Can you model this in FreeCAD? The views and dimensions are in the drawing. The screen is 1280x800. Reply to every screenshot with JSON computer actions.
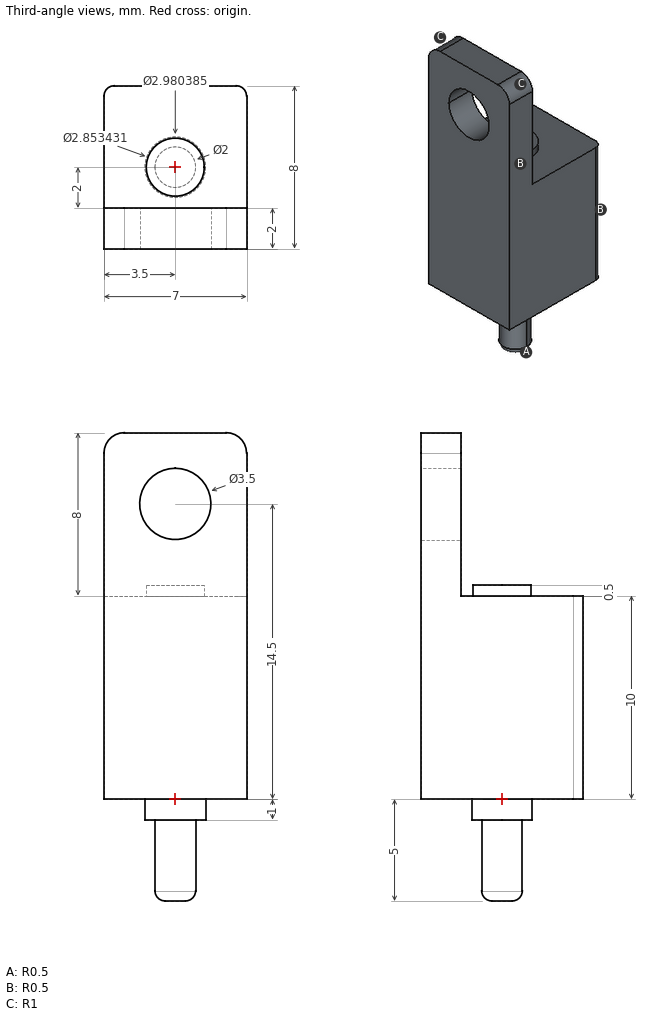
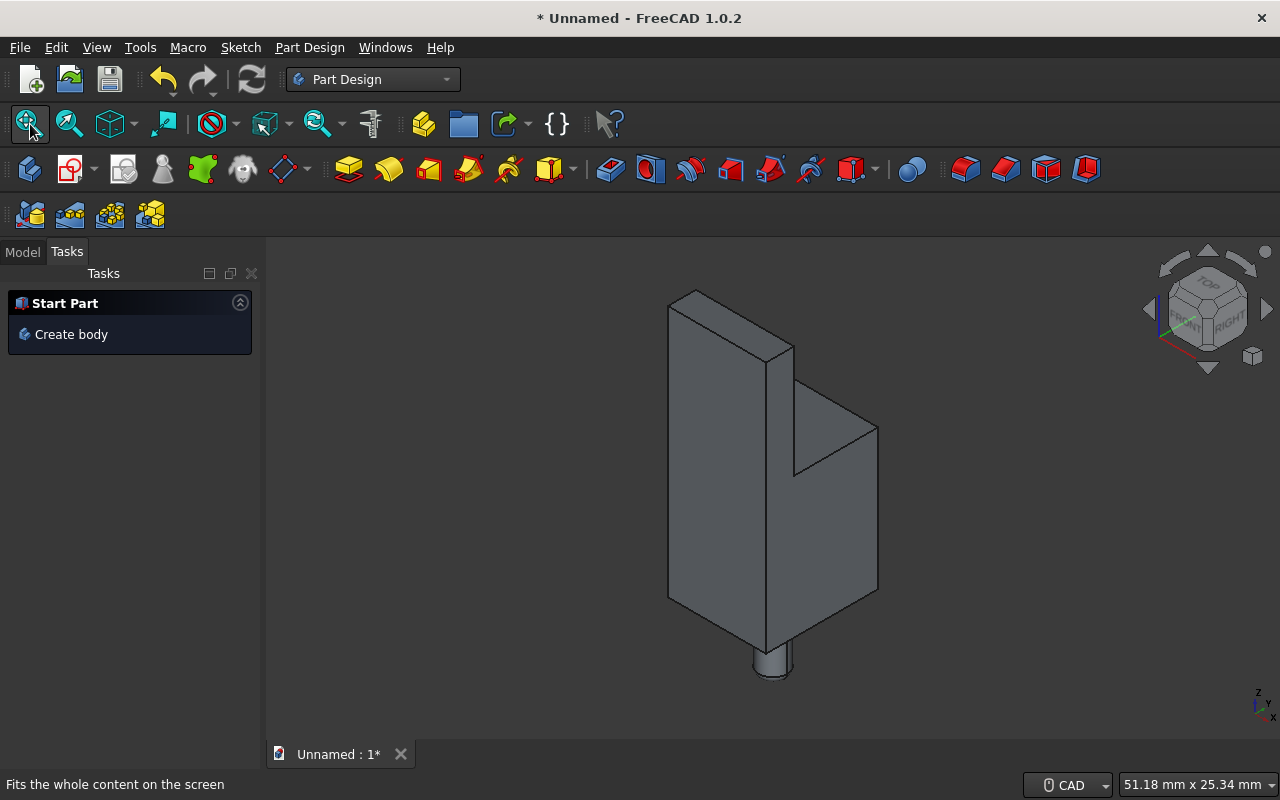
{"action": "left_click", "coordinate": [813, 423]}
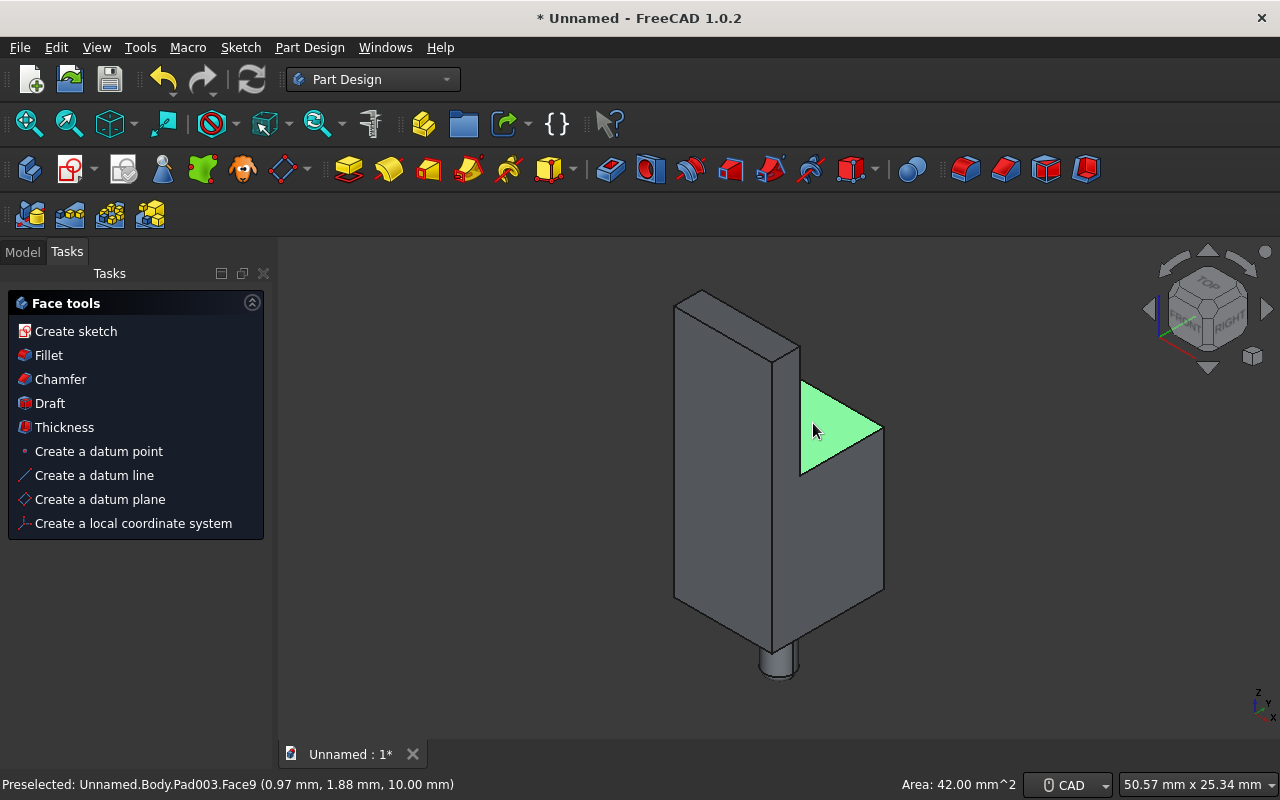
{"action": "left_click", "coordinate": [70, 170]}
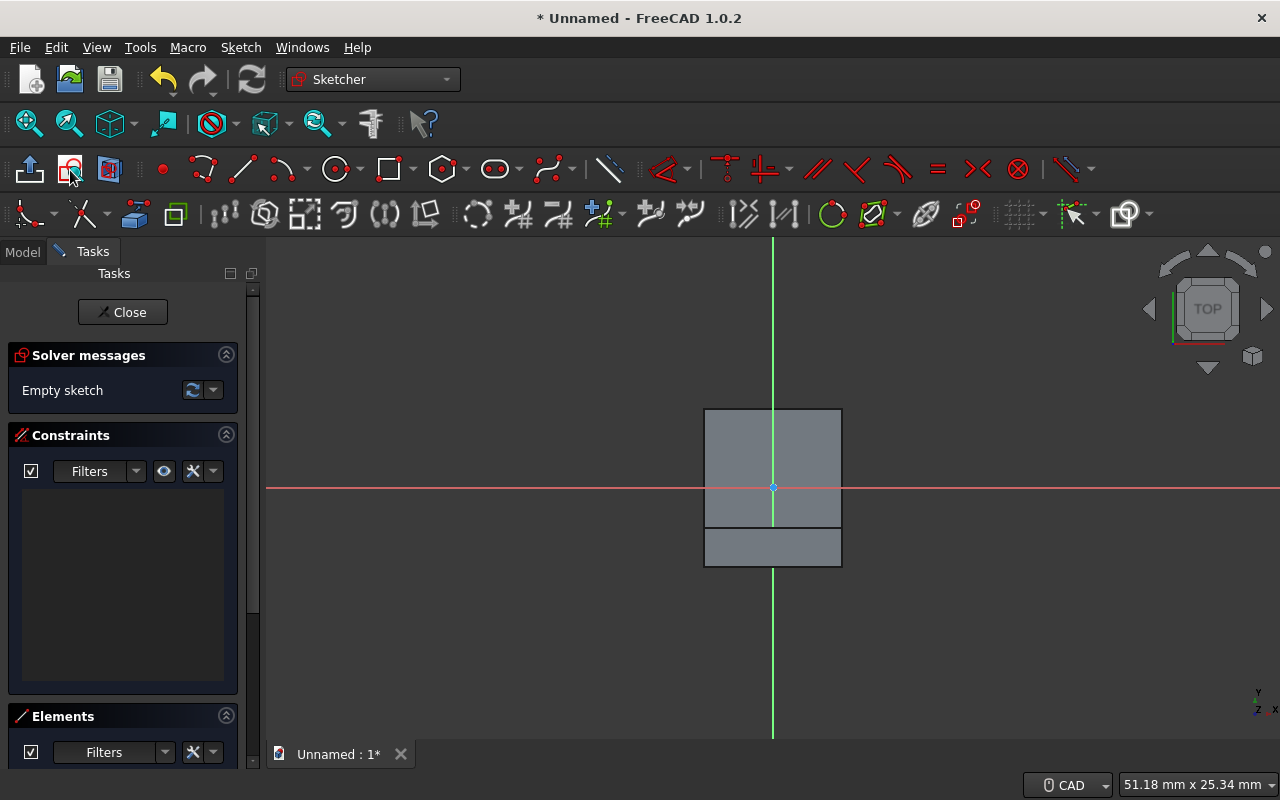
{"action": "key", "text": "q s"}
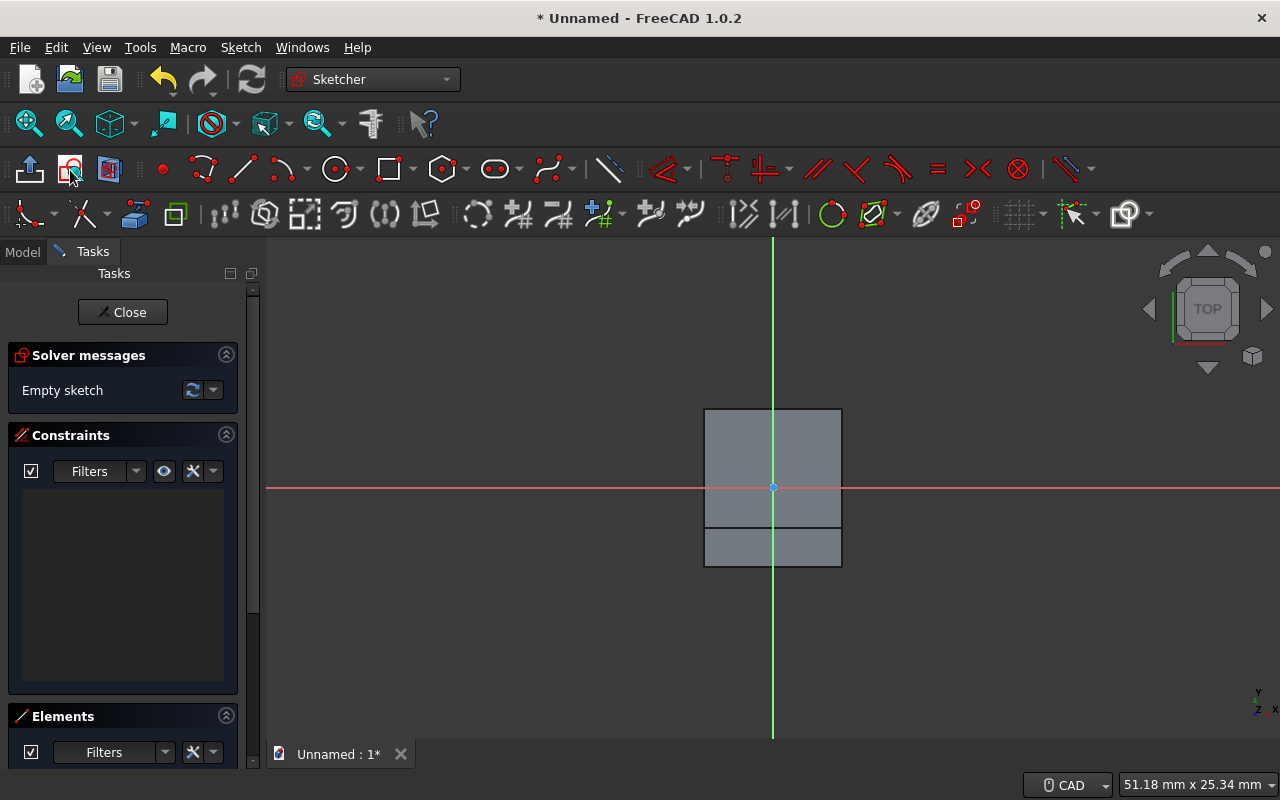
{"action": "scroll", "coordinate": [787, 488], "scroll_direction": "up", "scroll_amount": 9}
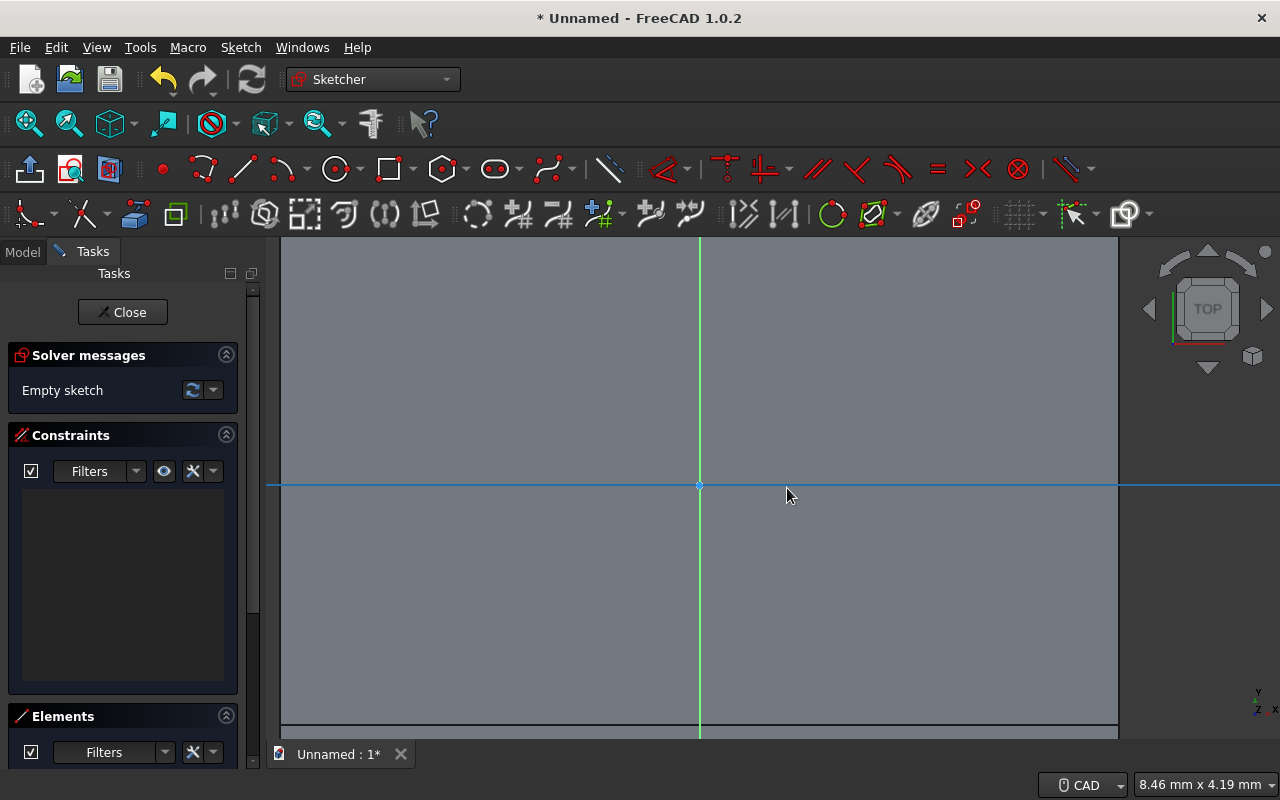
{"action": "left_click", "coordinate": [336, 170]}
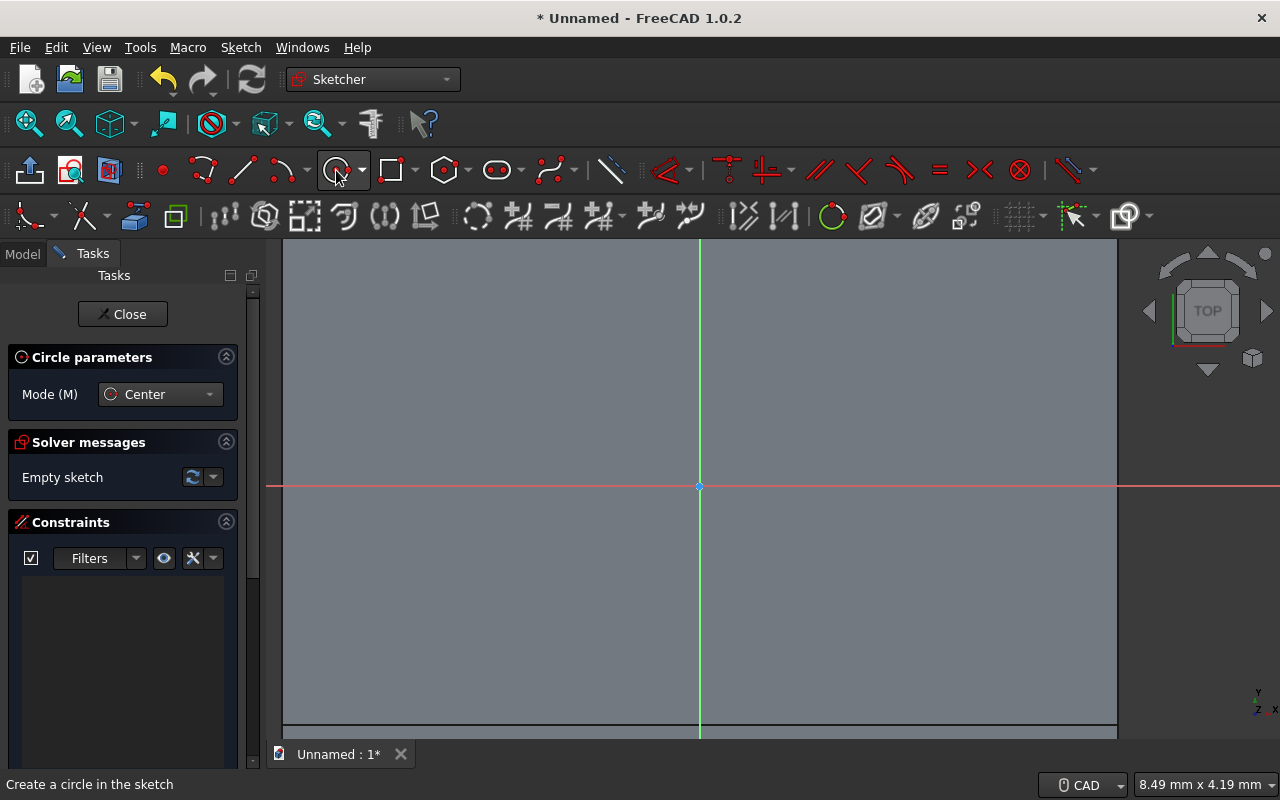
{"action": "left_click", "coordinate": [700, 486]}
{"action": "mouse_move", "coordinate": [820, 366]}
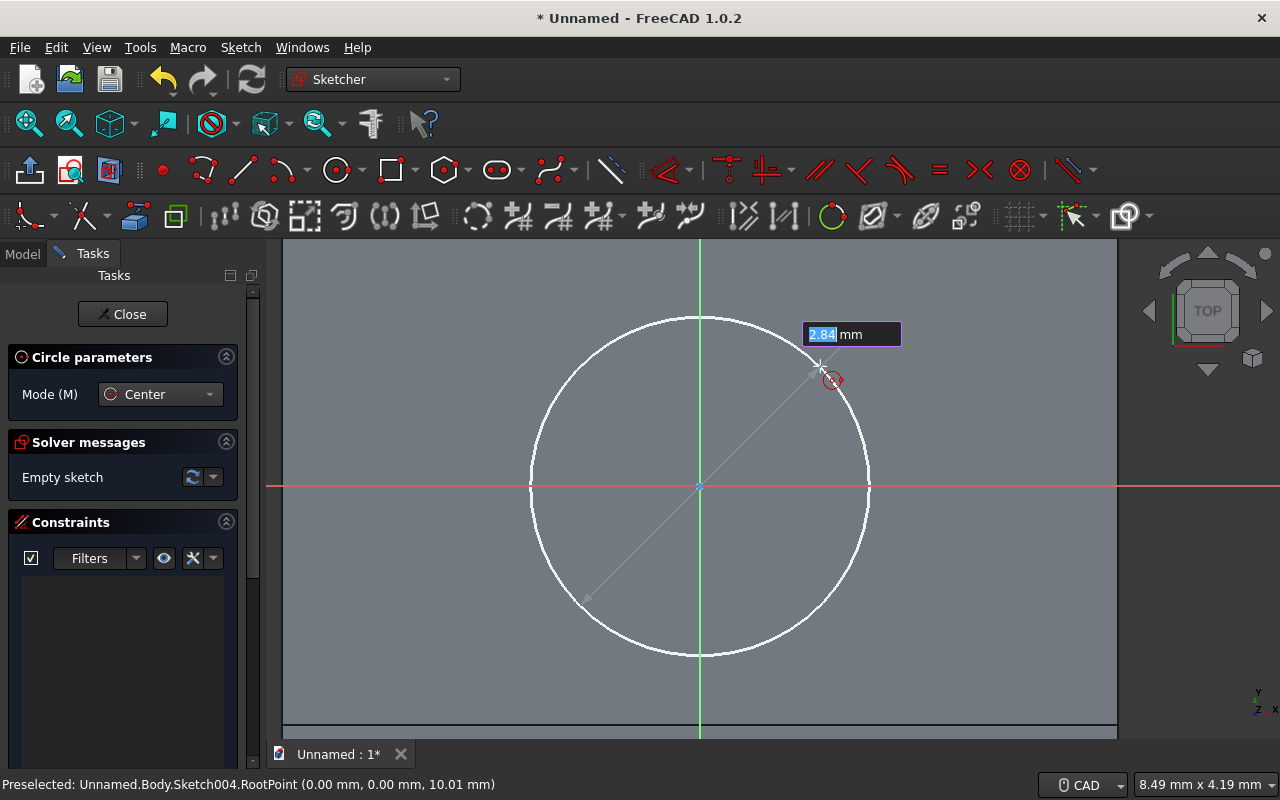
{"action": "type", "text": "2.853431"}
{"action": "key", "text": "Return"}
{"action": "key", "text": "Escape"}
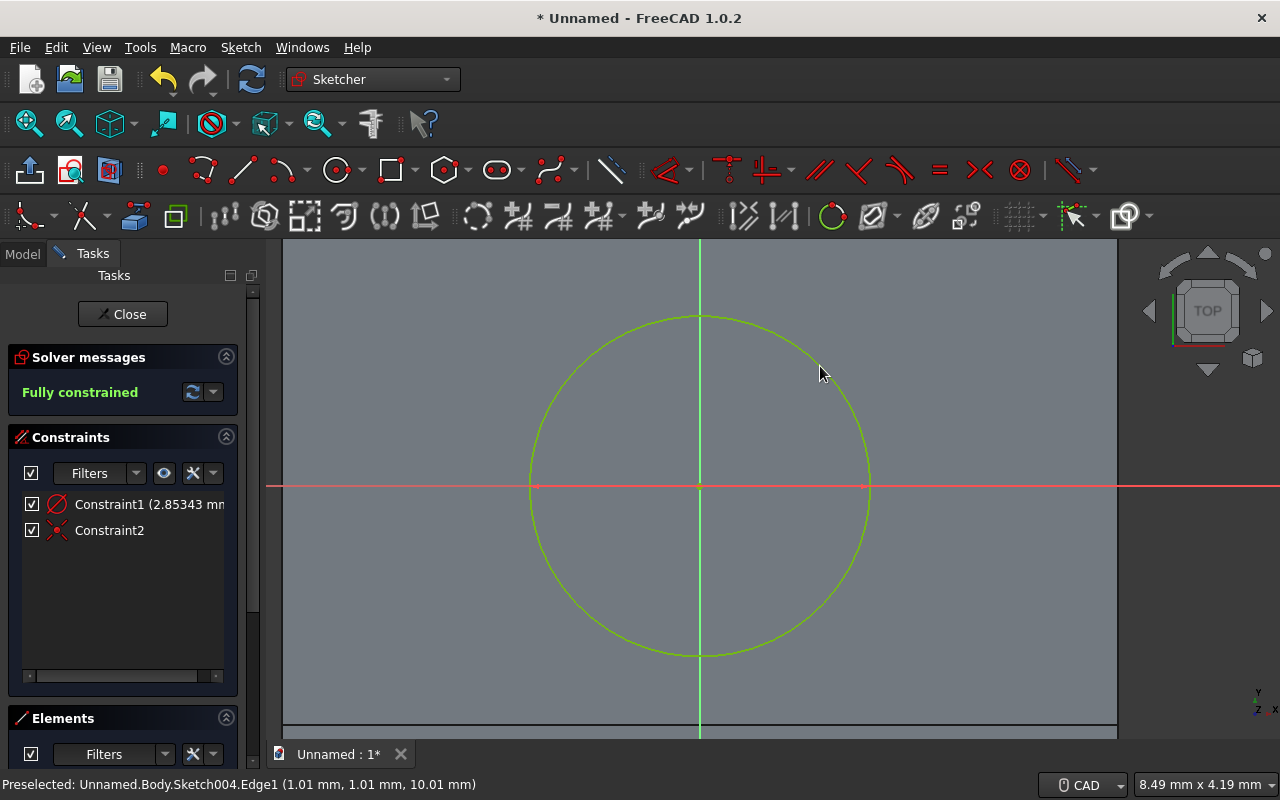
{"action": "left_click", "coordinate": [123, 314]}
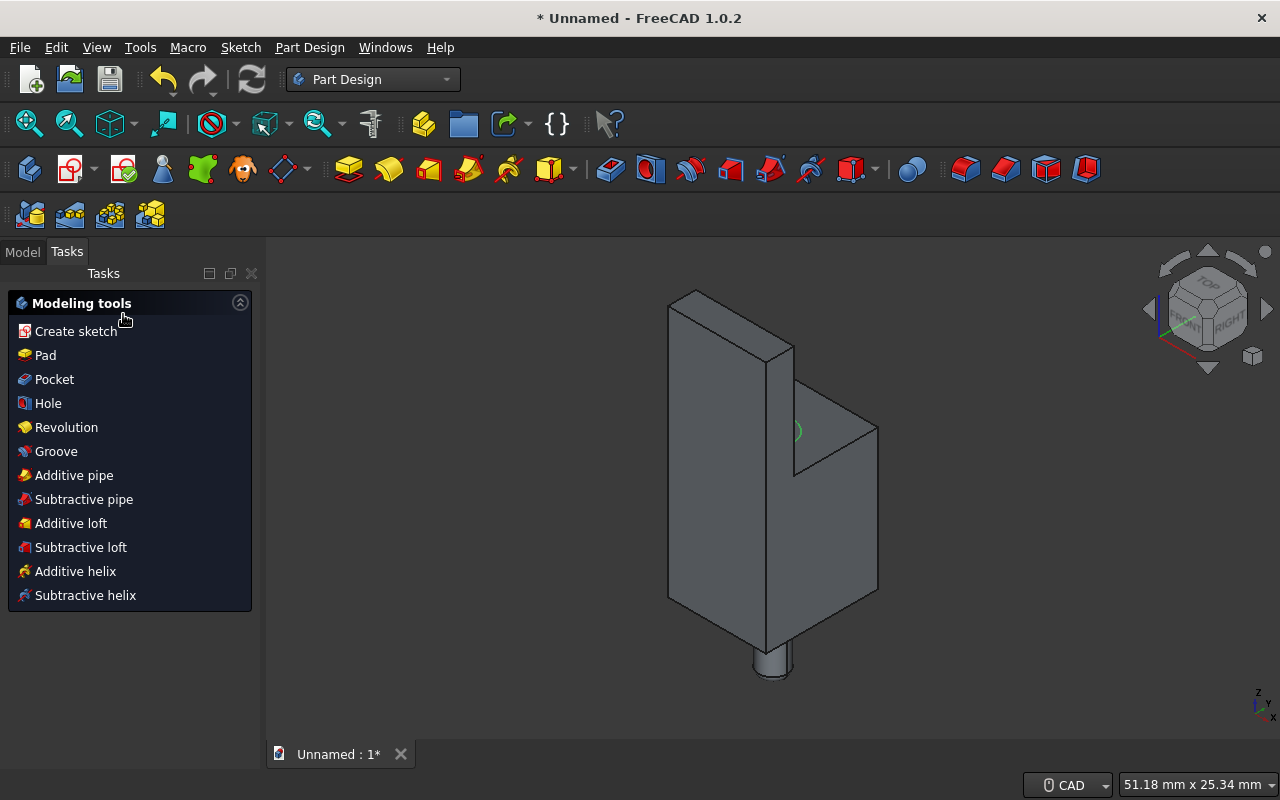
{"action": "left_click", "coordinate": [350, 170]}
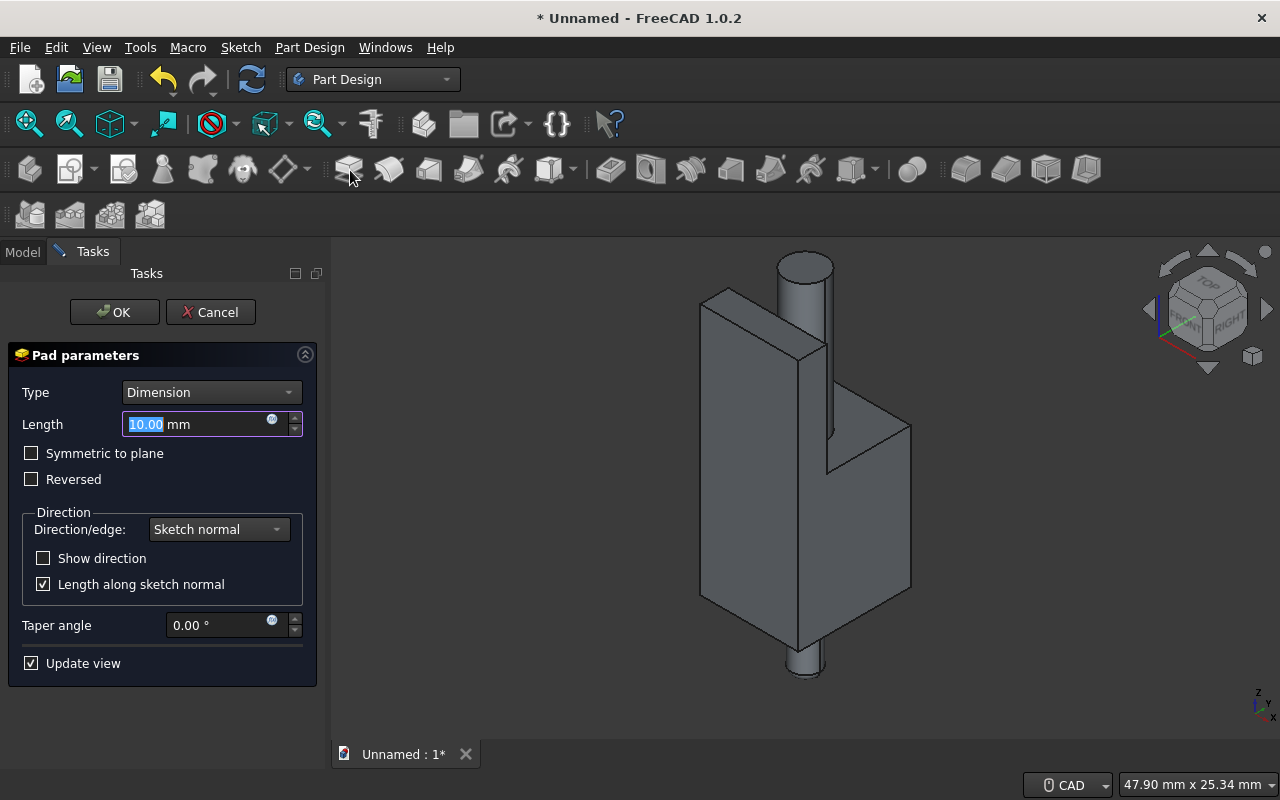
{"action": "type", "text": "0.5"}
{"action": "key", "text": "Tab"}